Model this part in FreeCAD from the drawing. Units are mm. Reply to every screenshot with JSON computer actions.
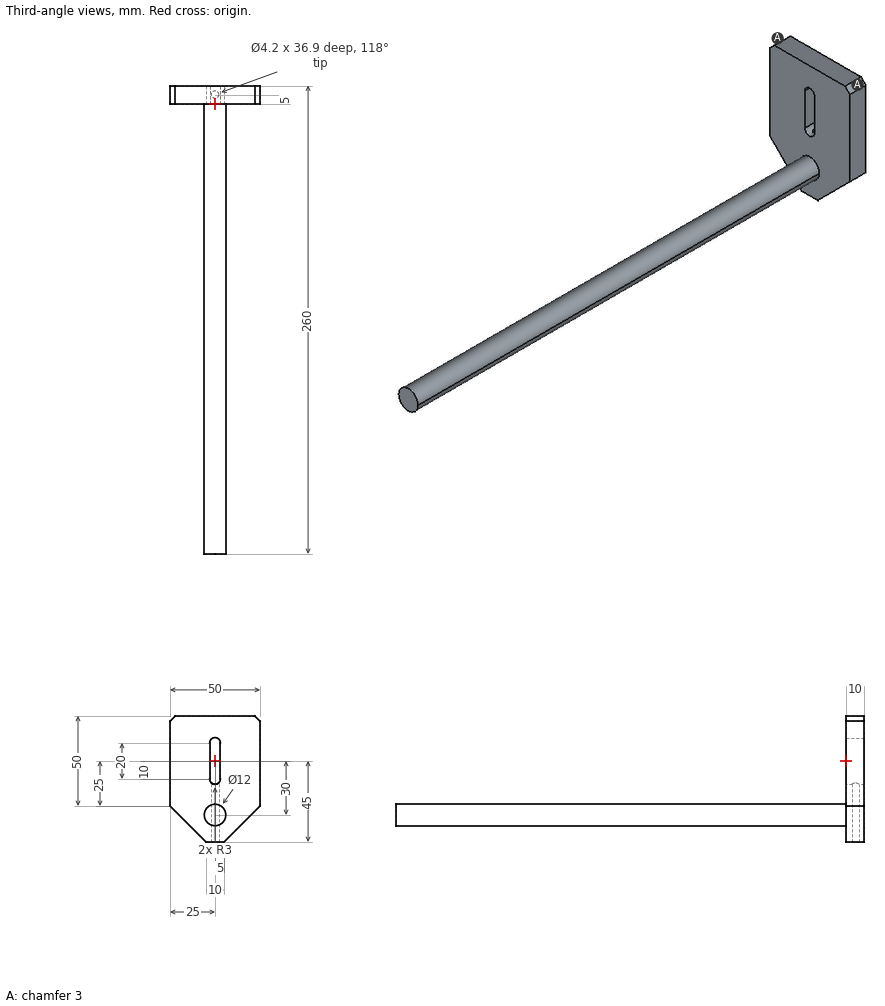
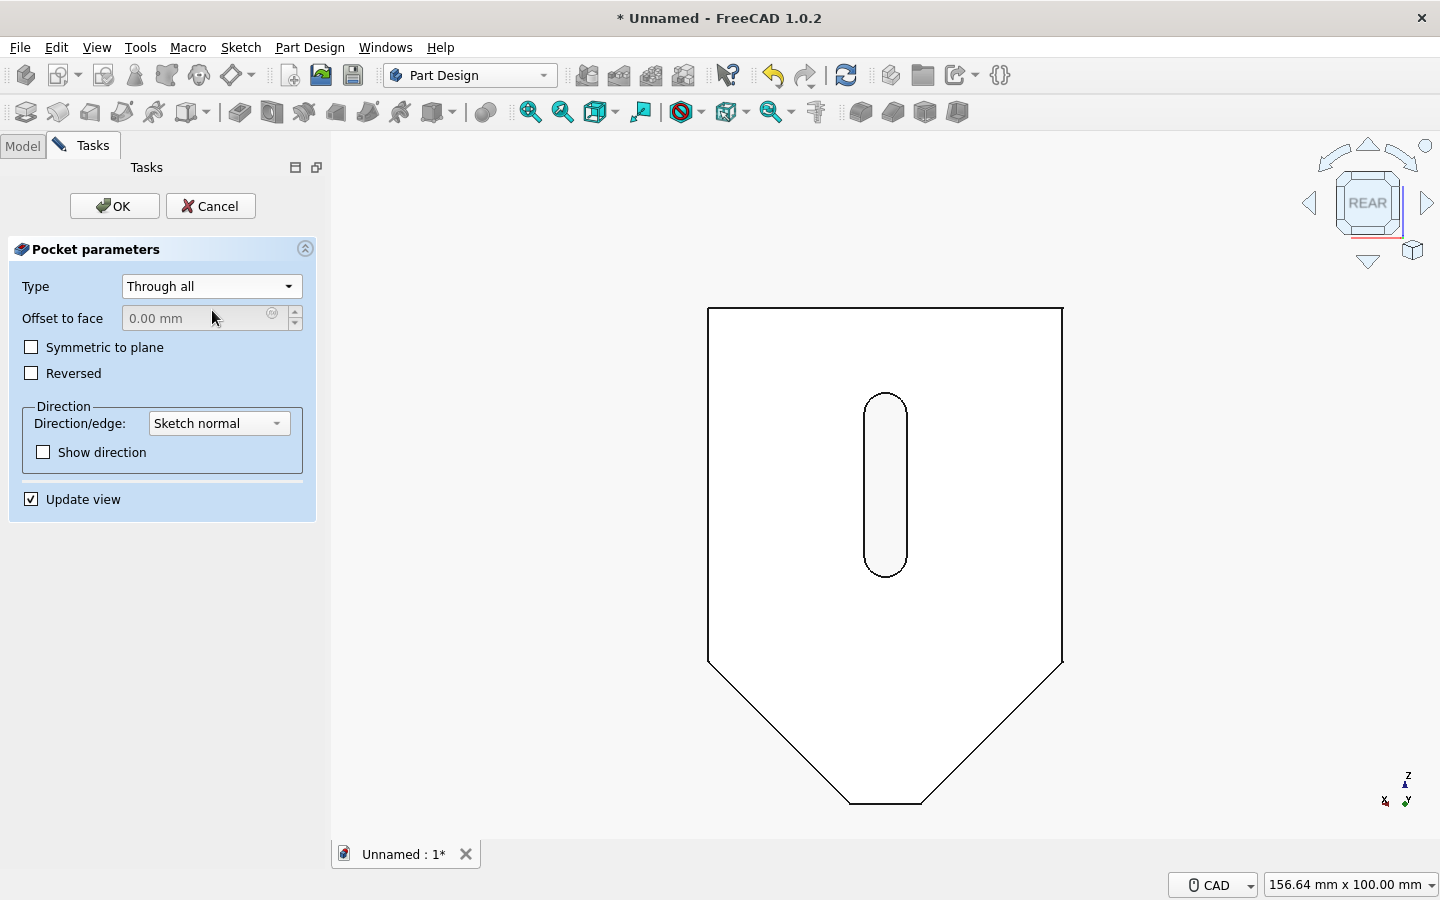
{"action": "left_click", "coordinate": [115, 206]}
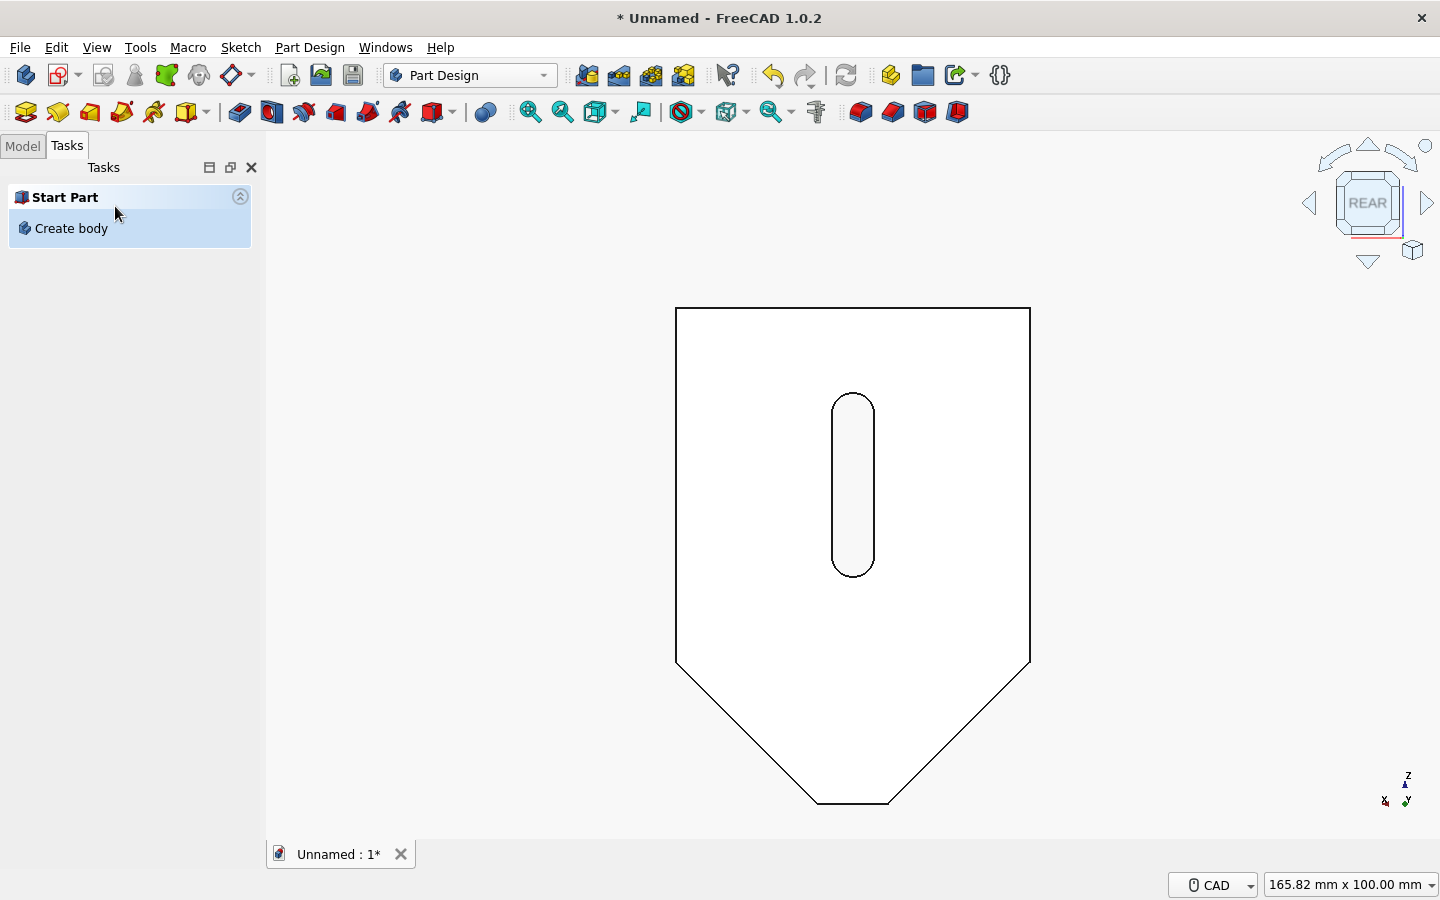
{"action": "key", "text": "5"}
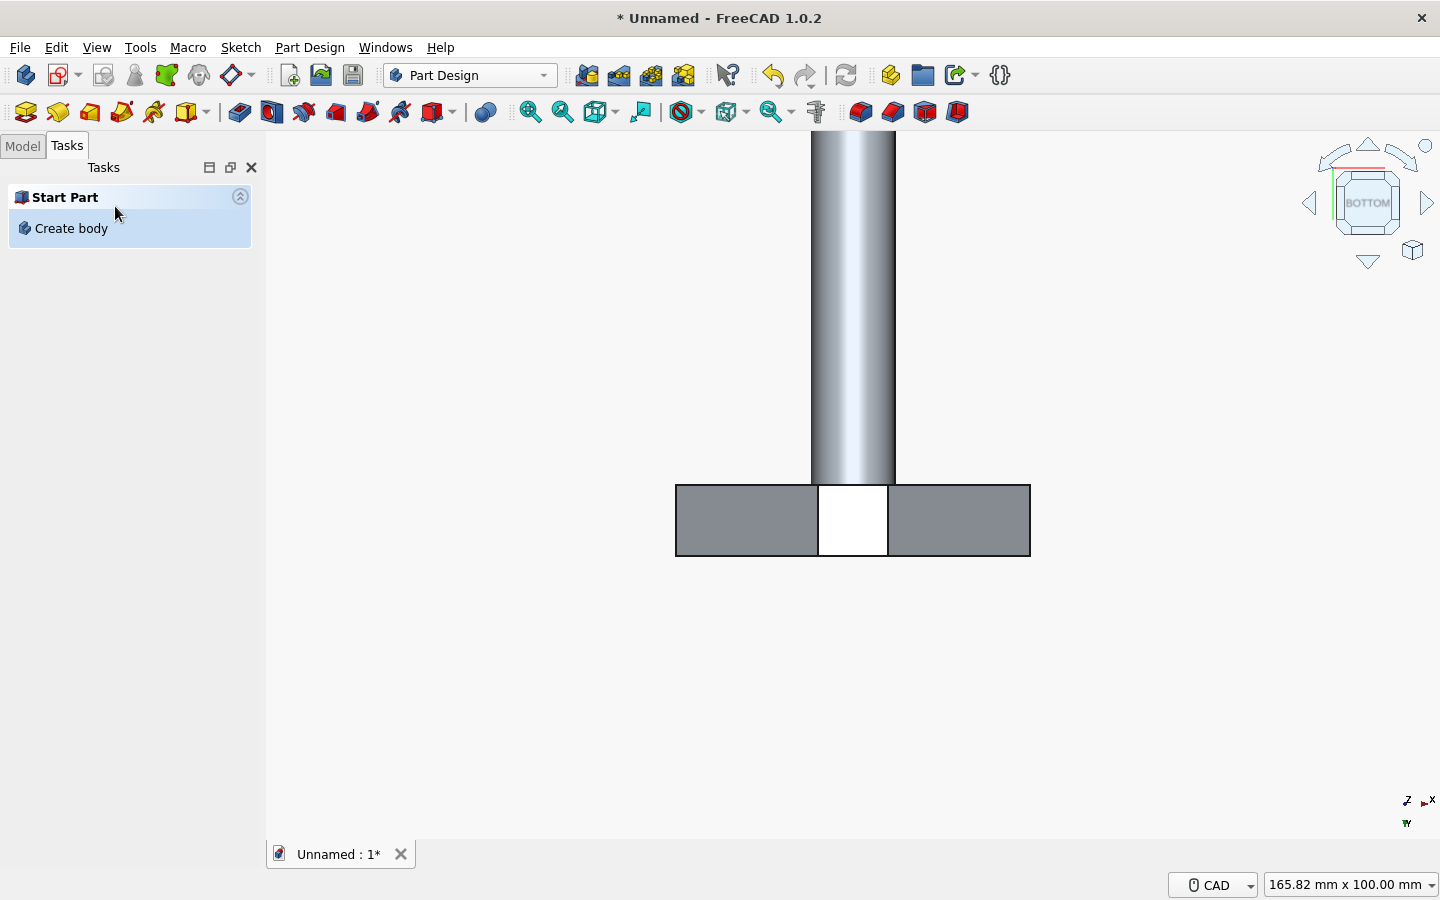
{"action": "left_click", "coordinate": [532, 112]}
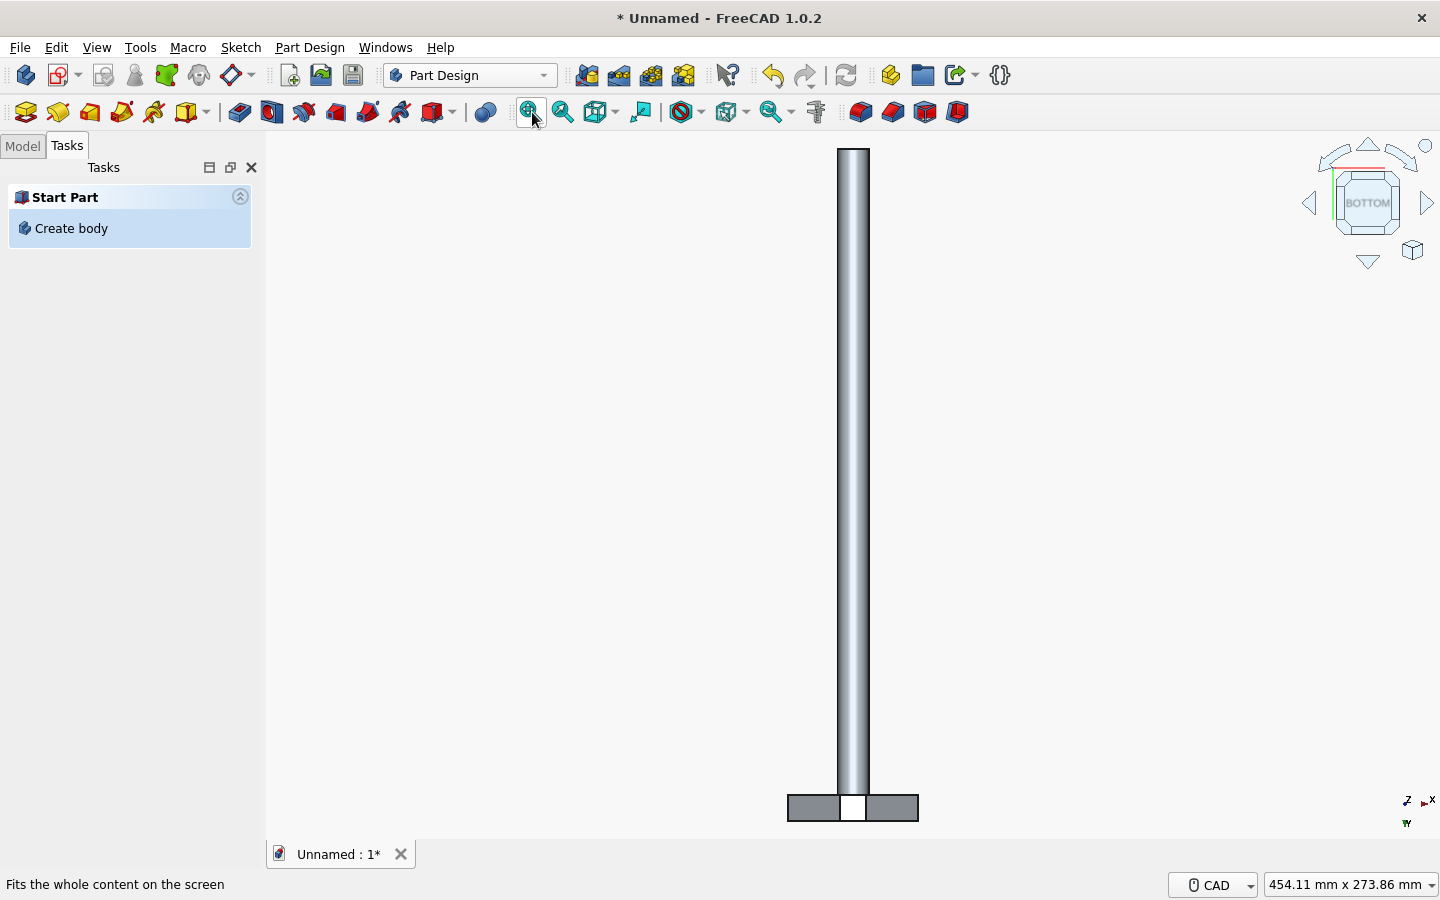
{"action": "left_click", "coordinate": [853, 807]}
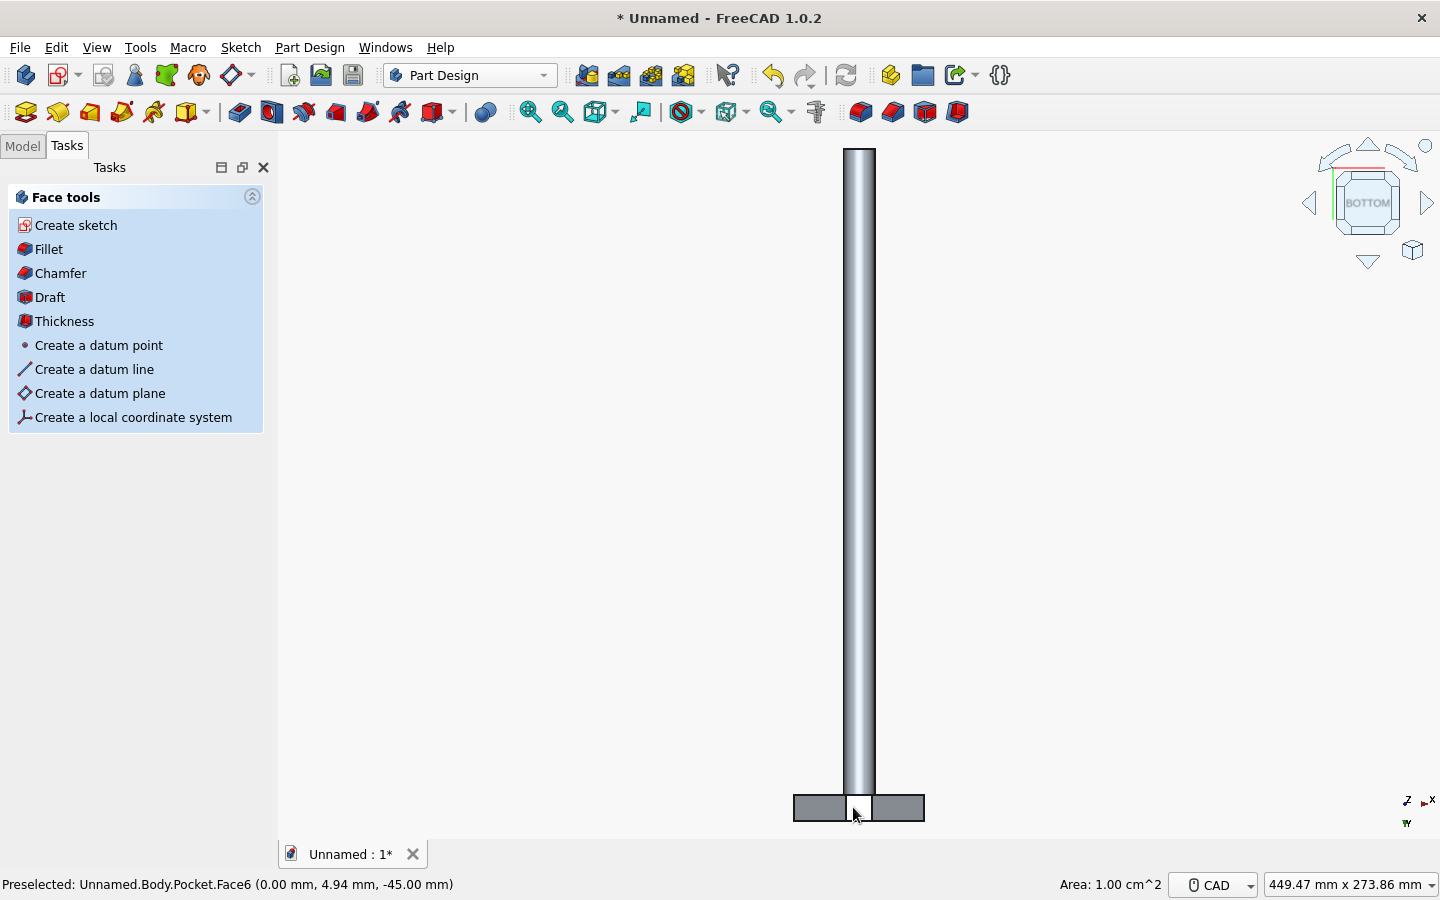
{"action": "left_click", "coordinate": [58, 76]}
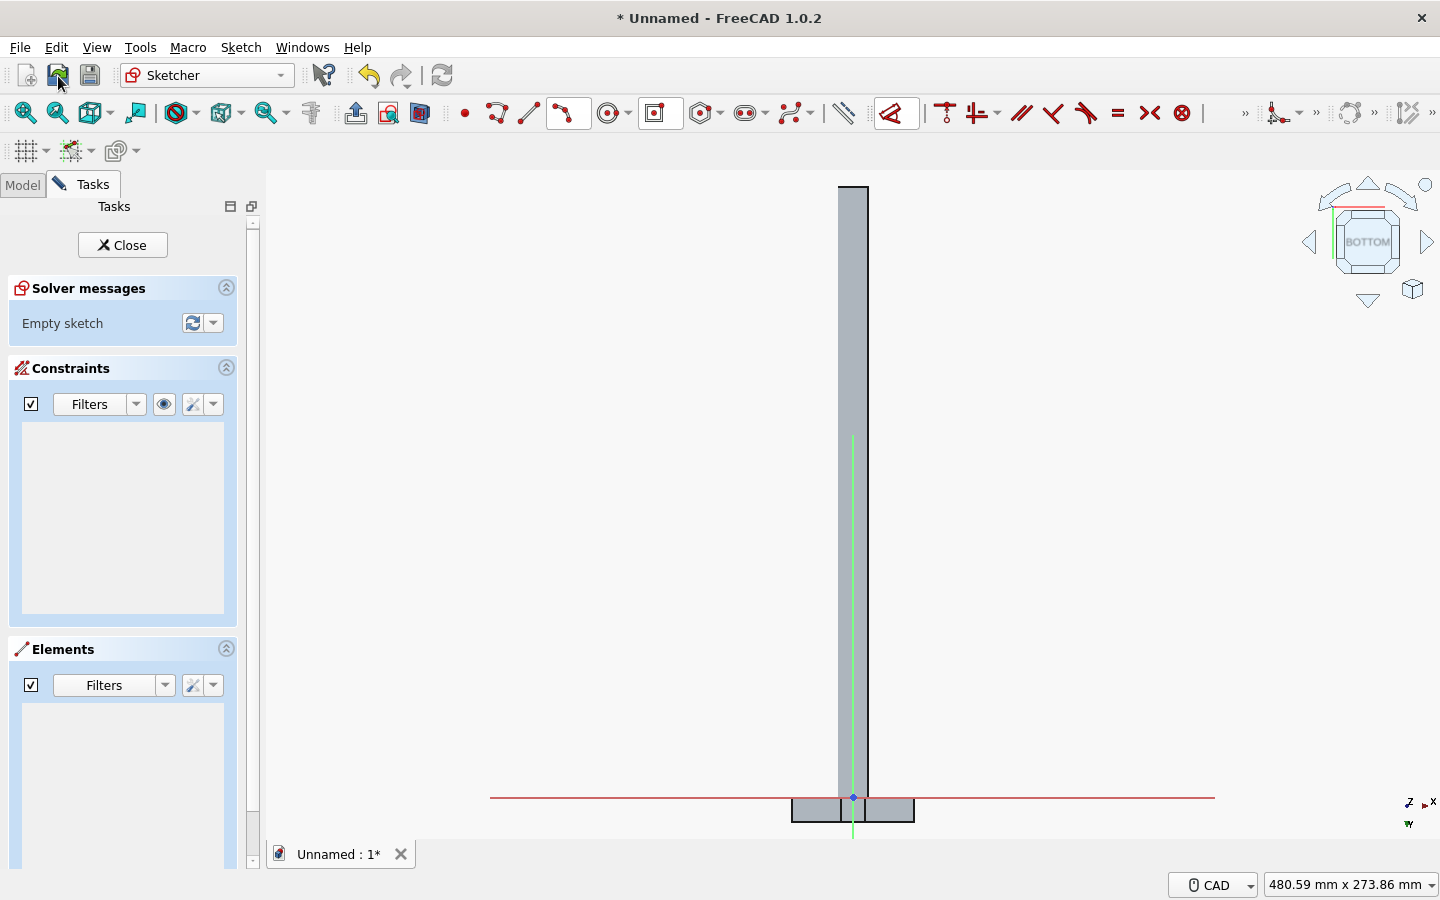
{"action": "scroll", "coordinate": [784, 504], "scroll_direction": "down", "scroll_amount": 5}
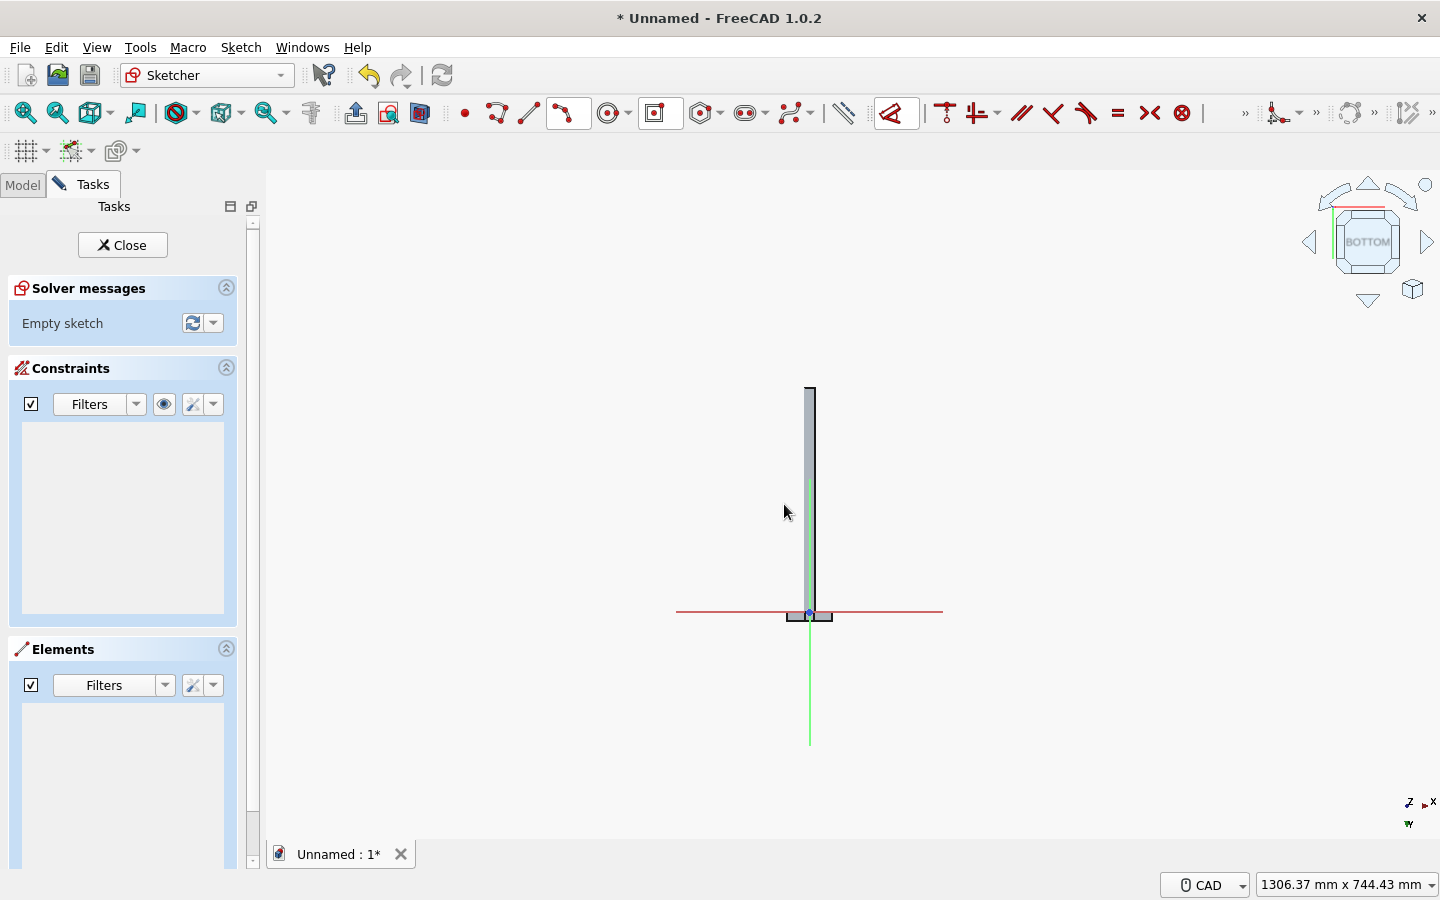
{"action": "scroll", "coordinate": [811, 621], "scroll_direction": "up", "scroll_amount": 15}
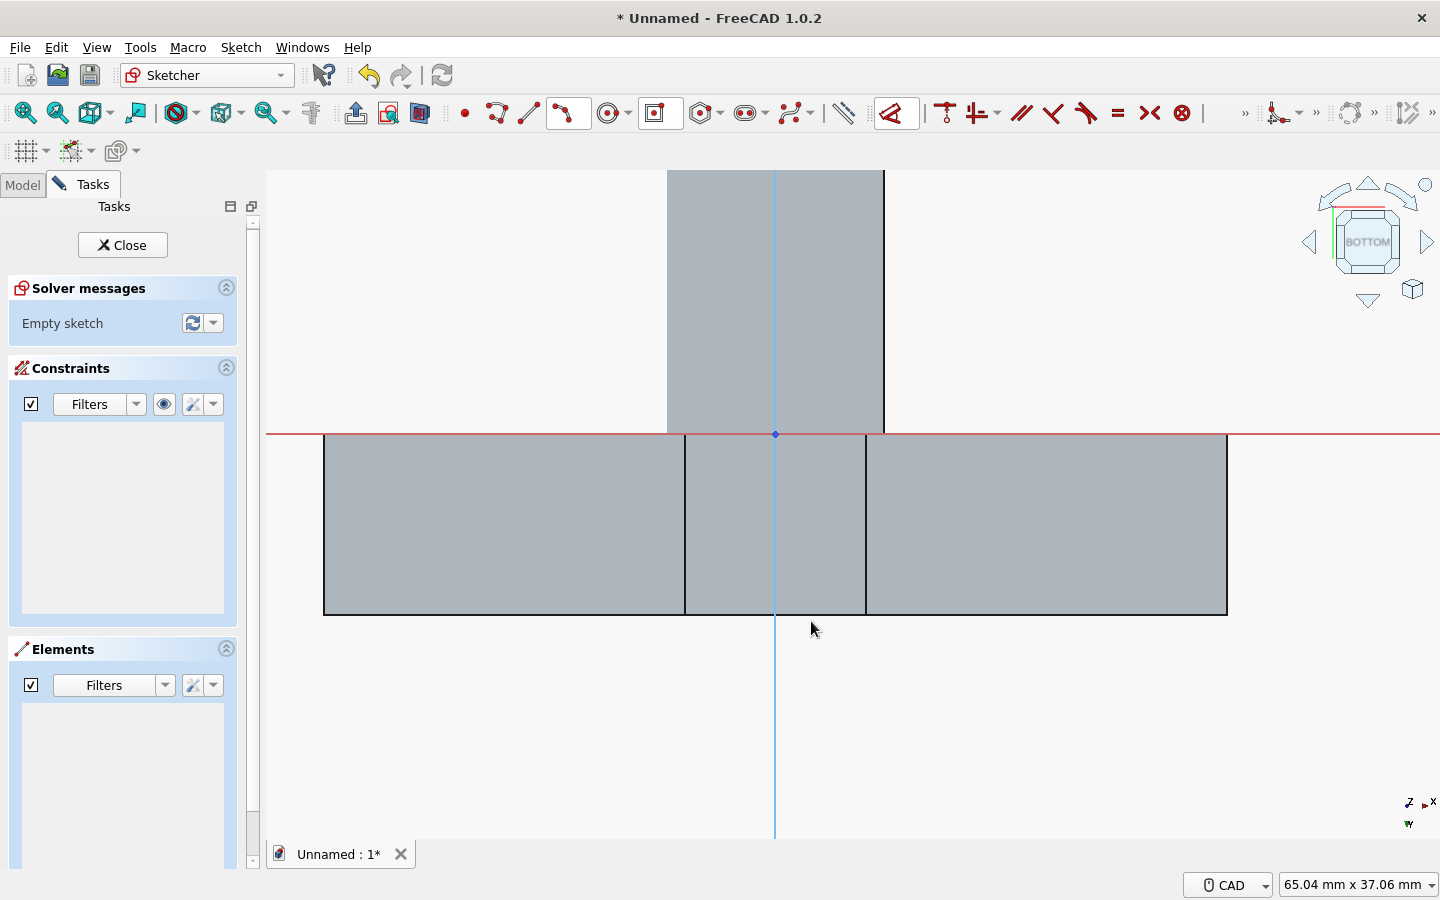
{"action": "scroll", "coordinate": [771, 496], "scroll_direction": "up", "scroll_amount": 6}